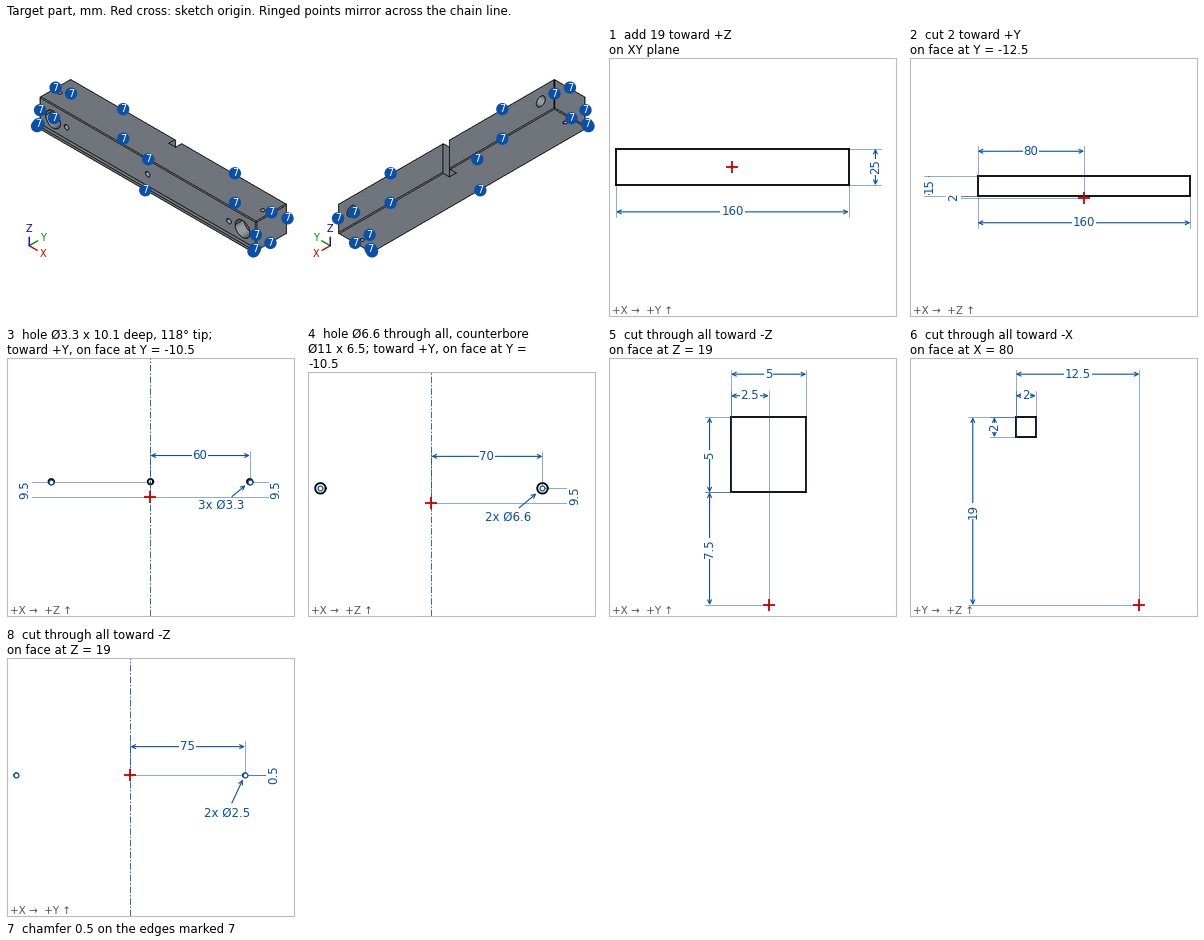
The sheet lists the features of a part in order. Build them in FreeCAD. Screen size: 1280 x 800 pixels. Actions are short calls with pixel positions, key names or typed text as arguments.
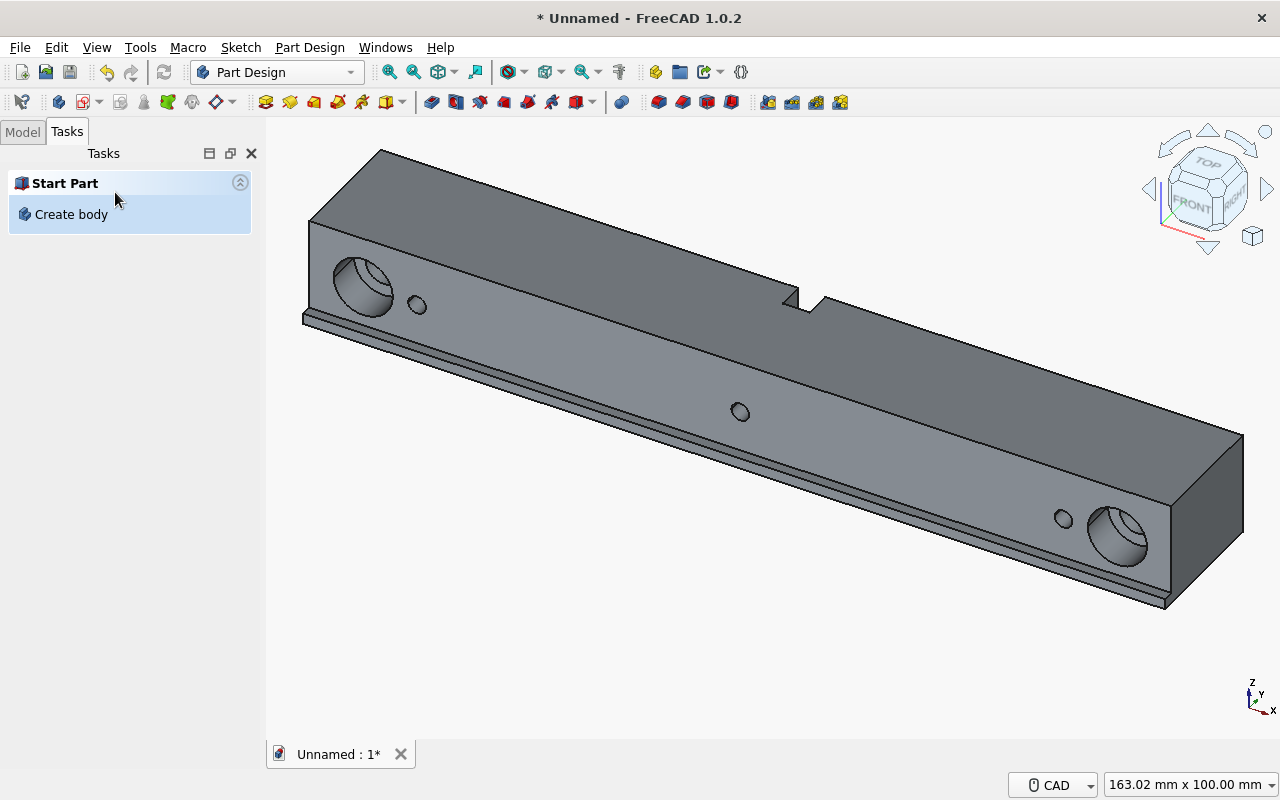
click(1204, 521)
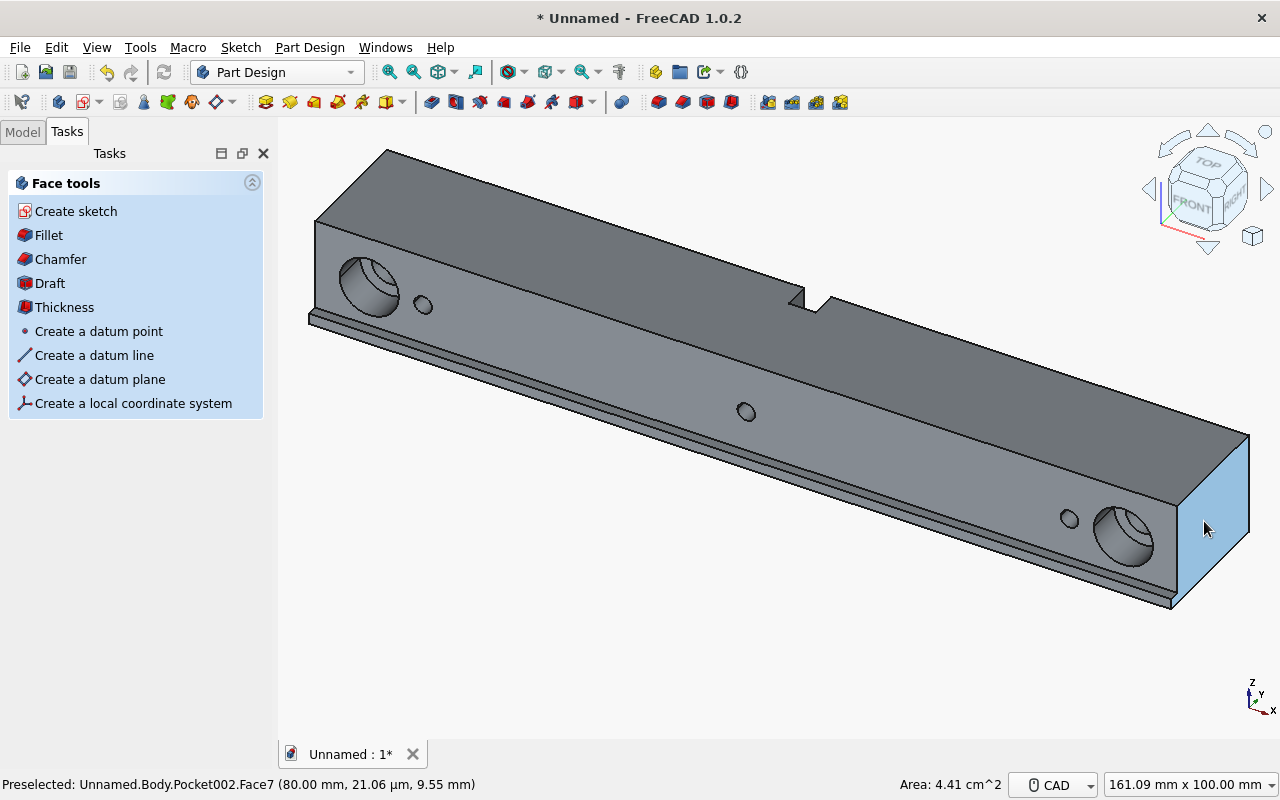
click(746, 363, ctrl)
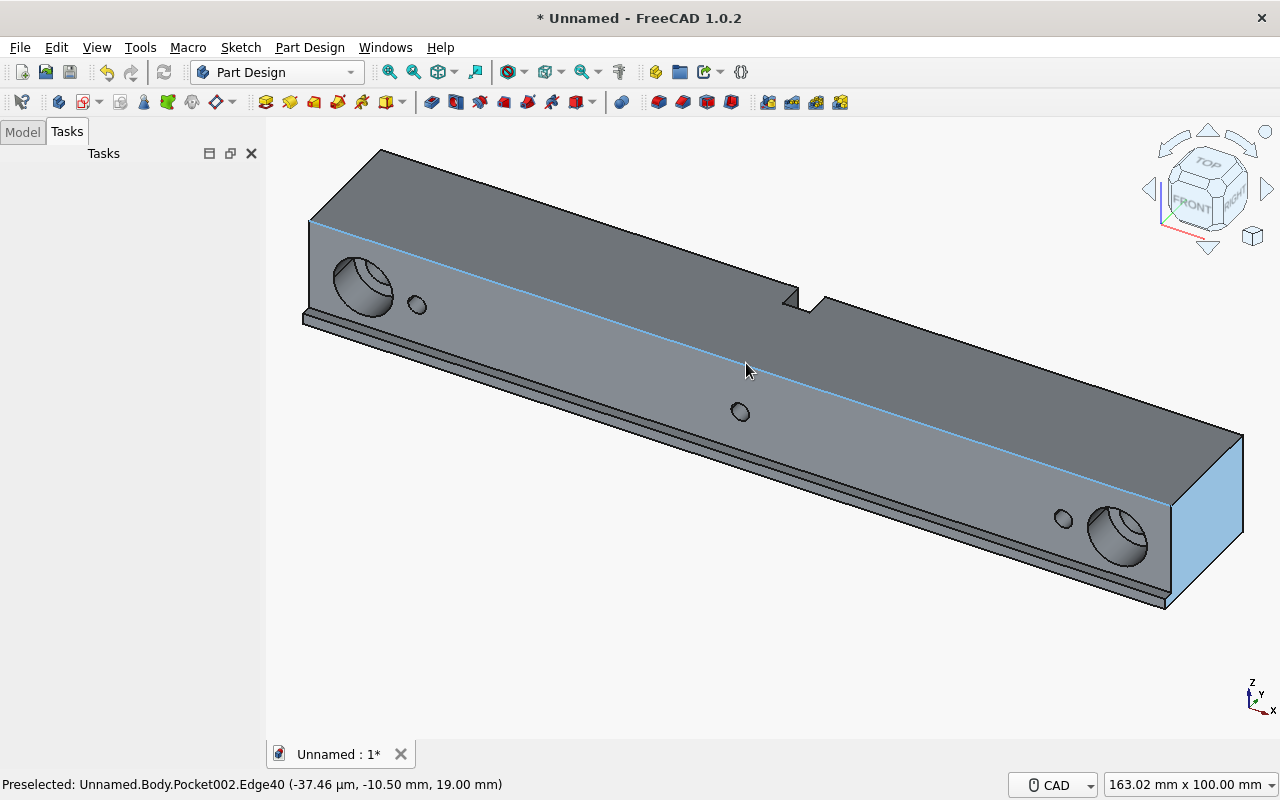
key(0)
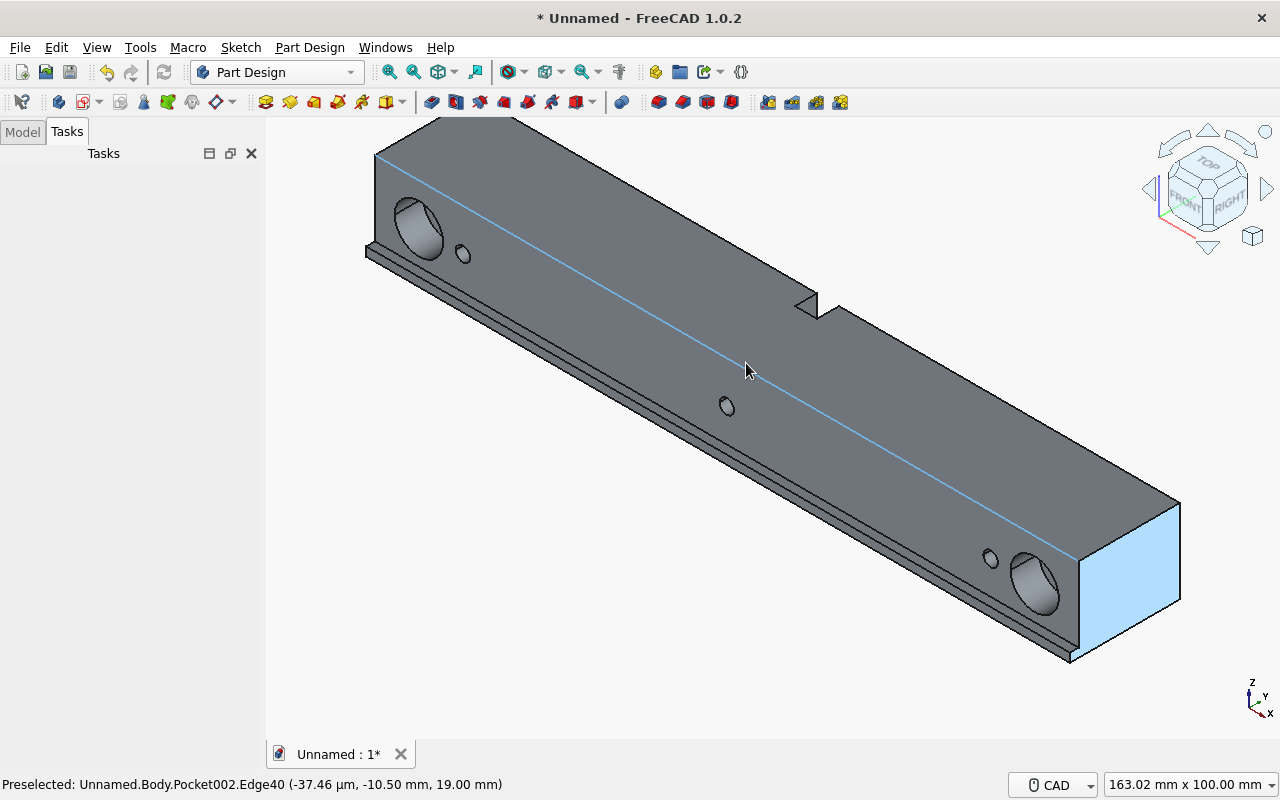
click(390, 72)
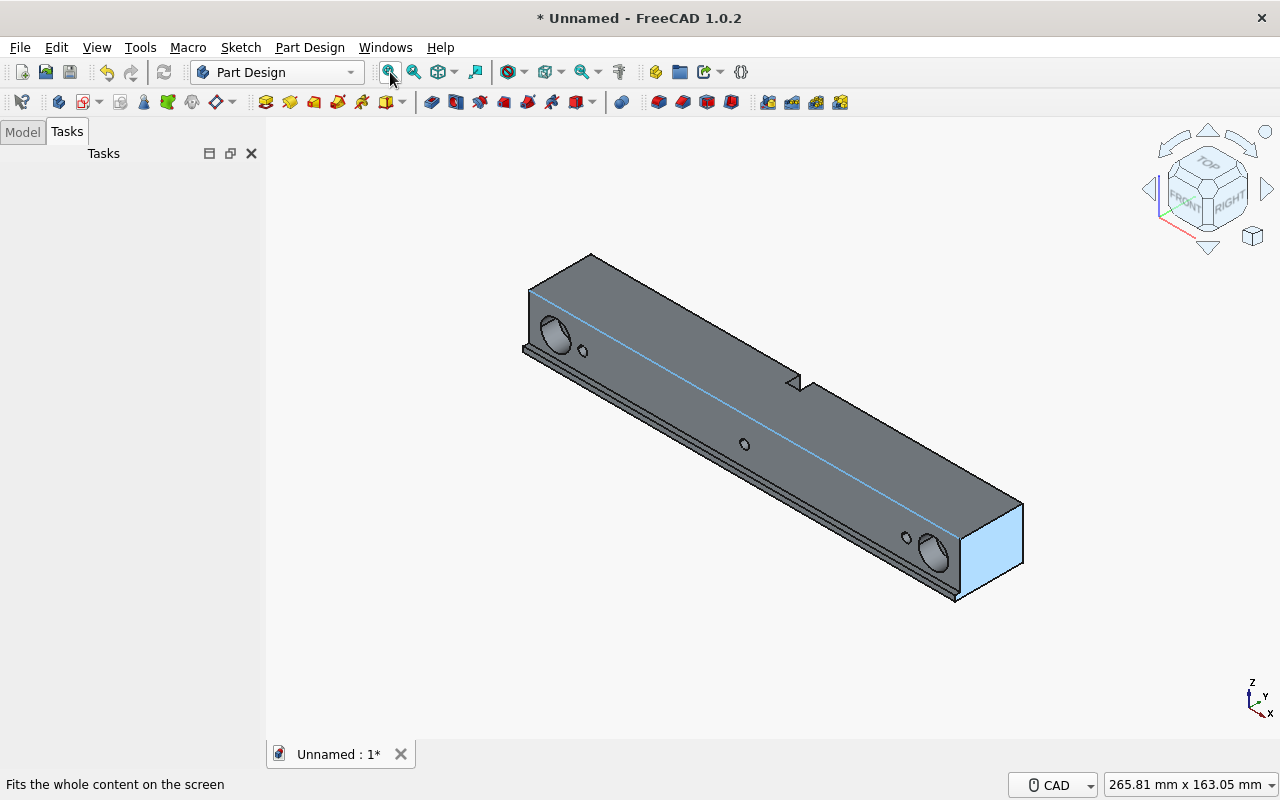
key(2)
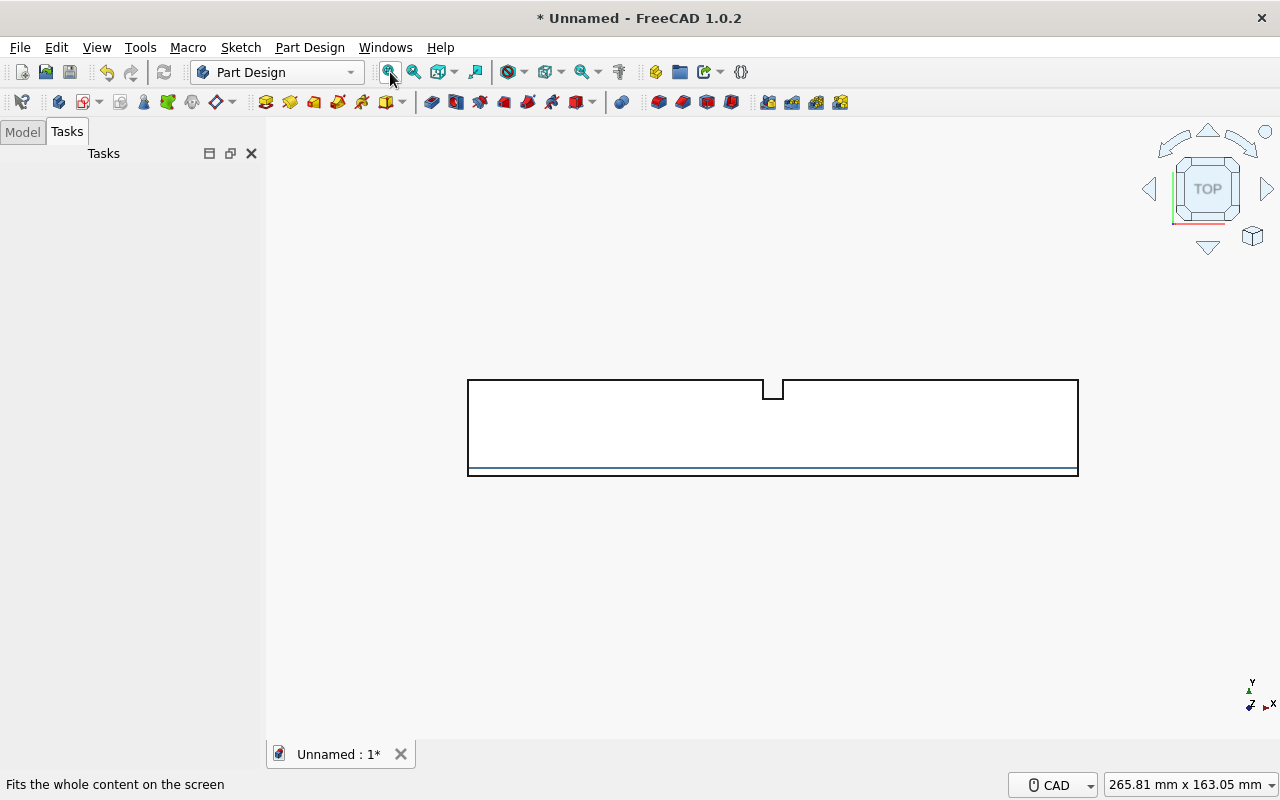
click(616, 379, ctrl)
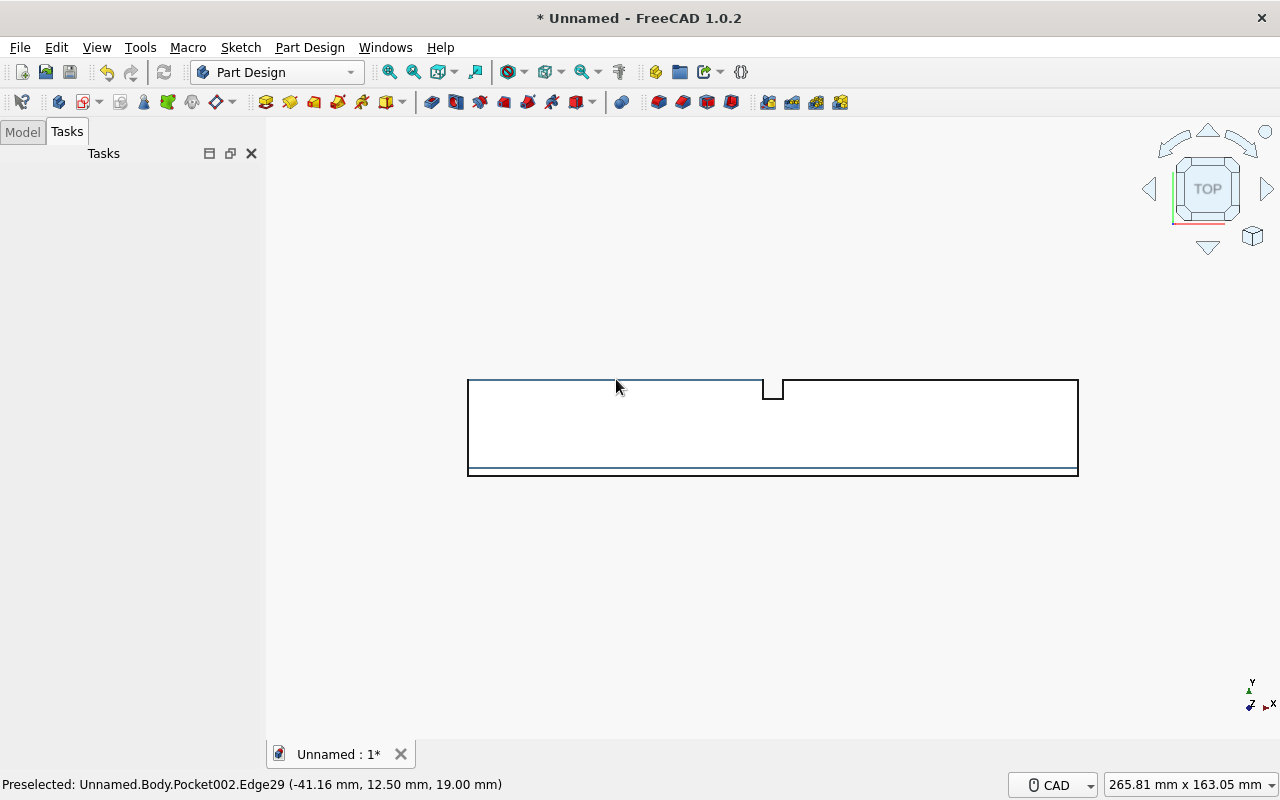
click(930, 379, ctrl)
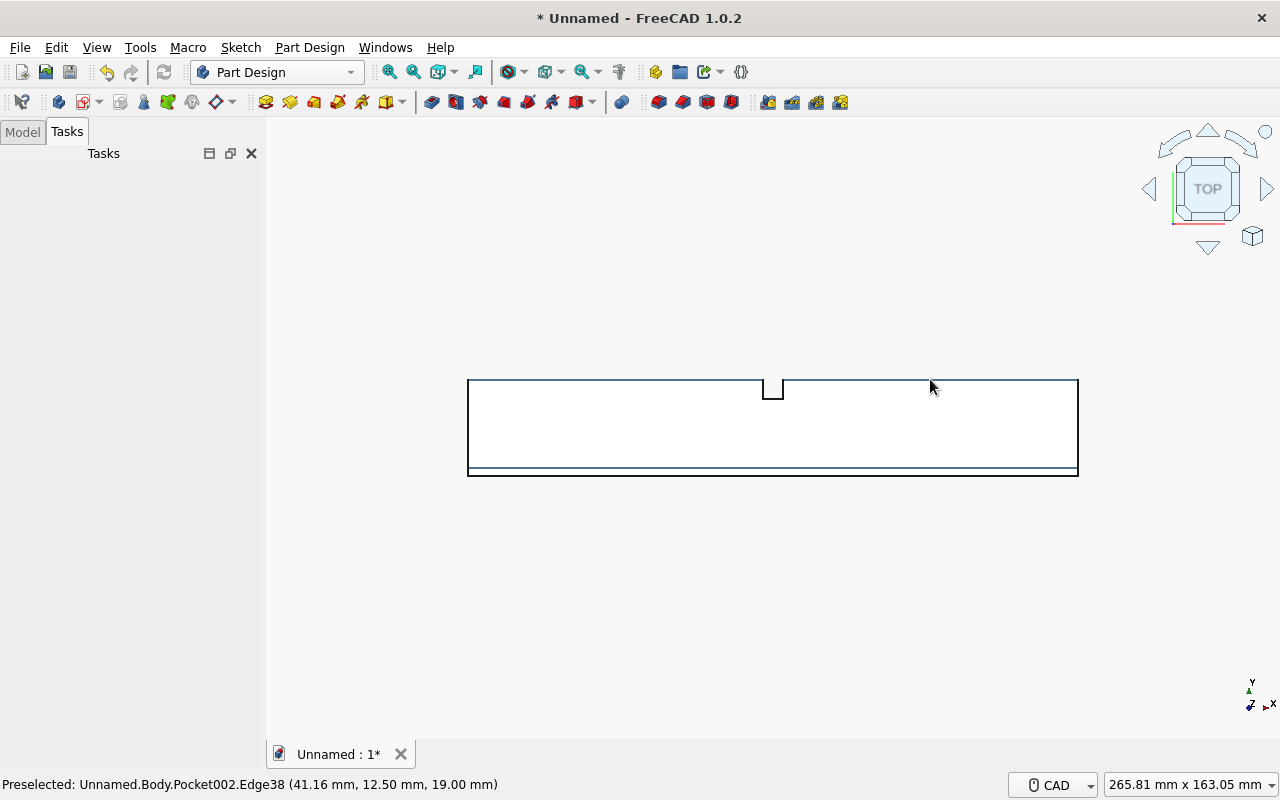
key(1)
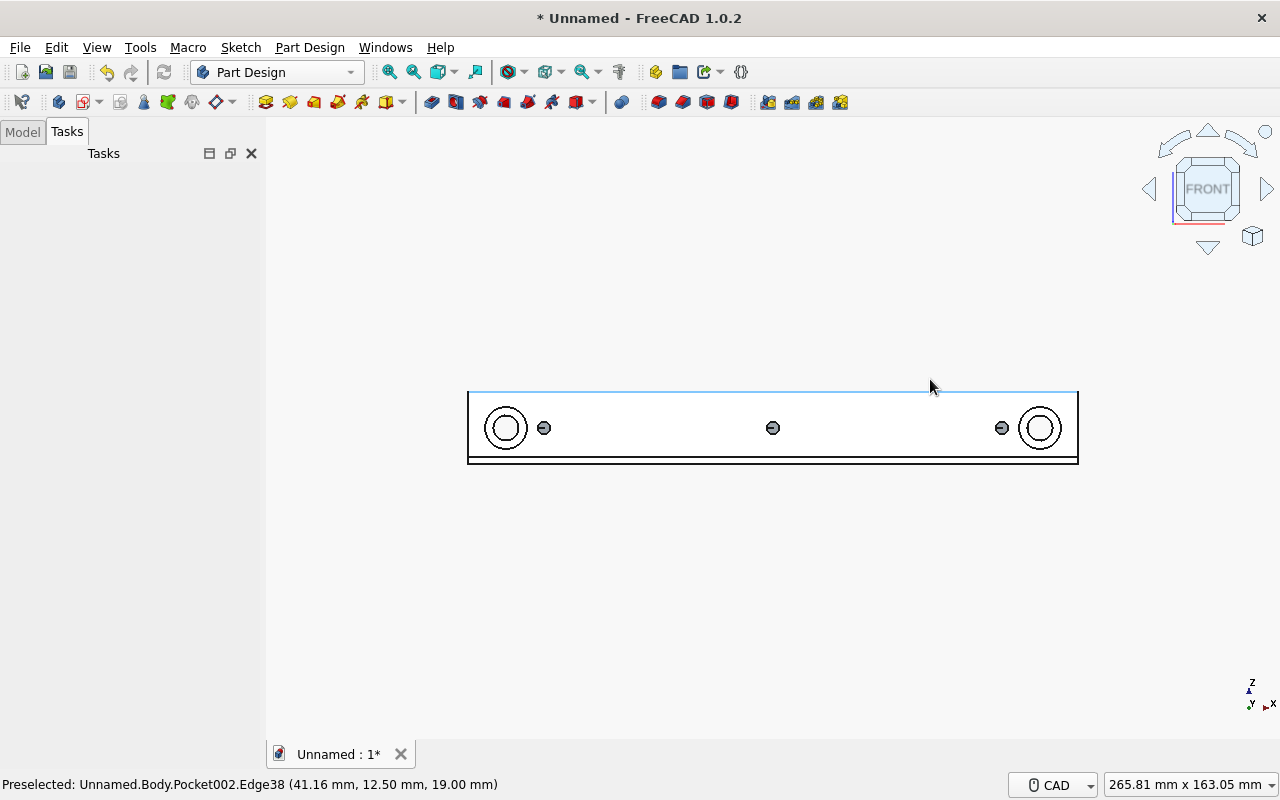
click(773, 463, ctrl)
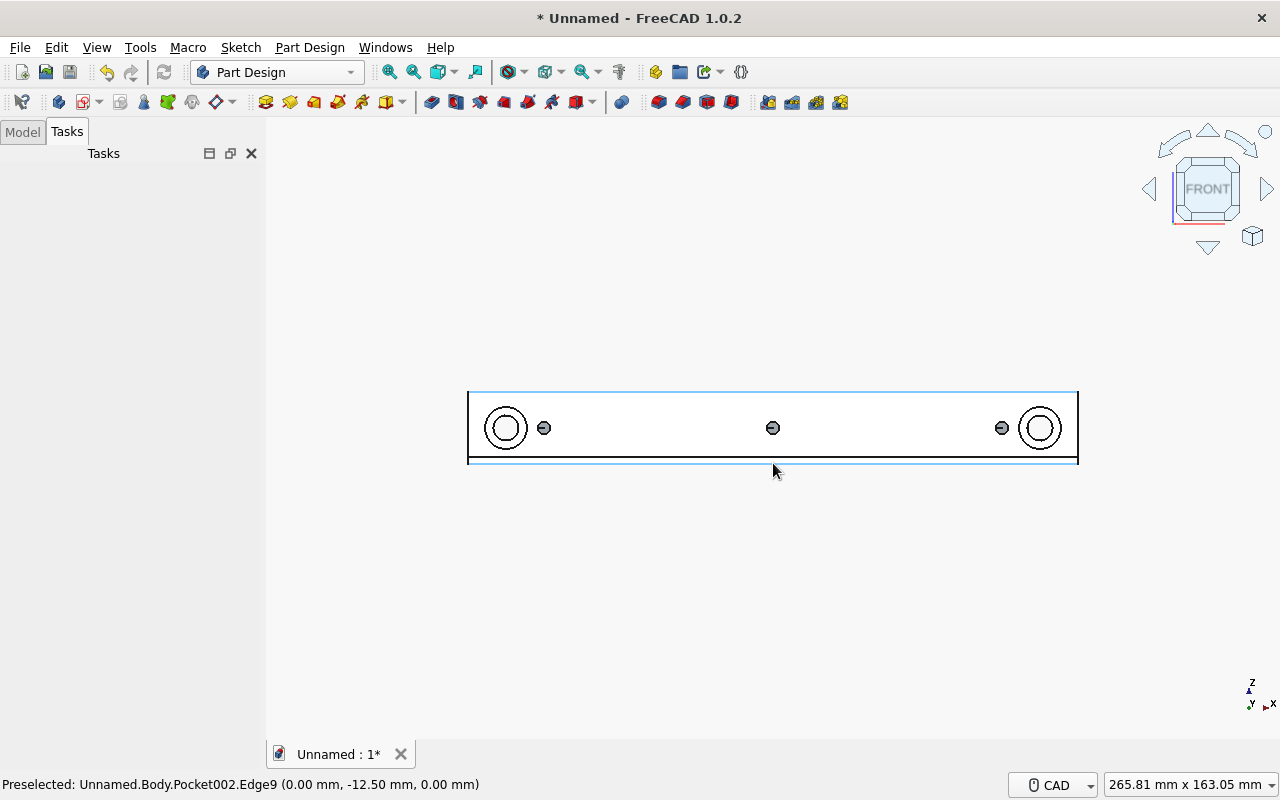
key(3)